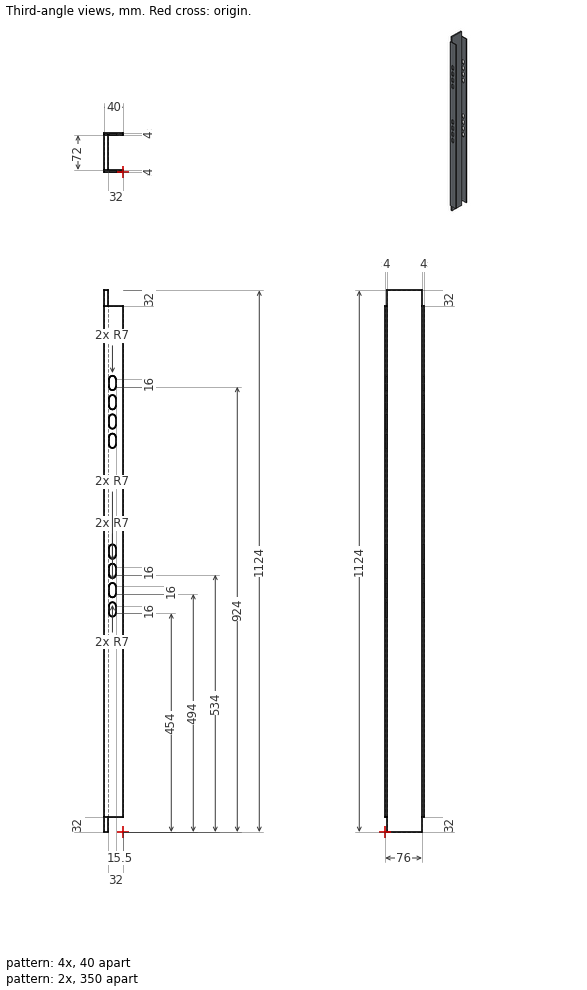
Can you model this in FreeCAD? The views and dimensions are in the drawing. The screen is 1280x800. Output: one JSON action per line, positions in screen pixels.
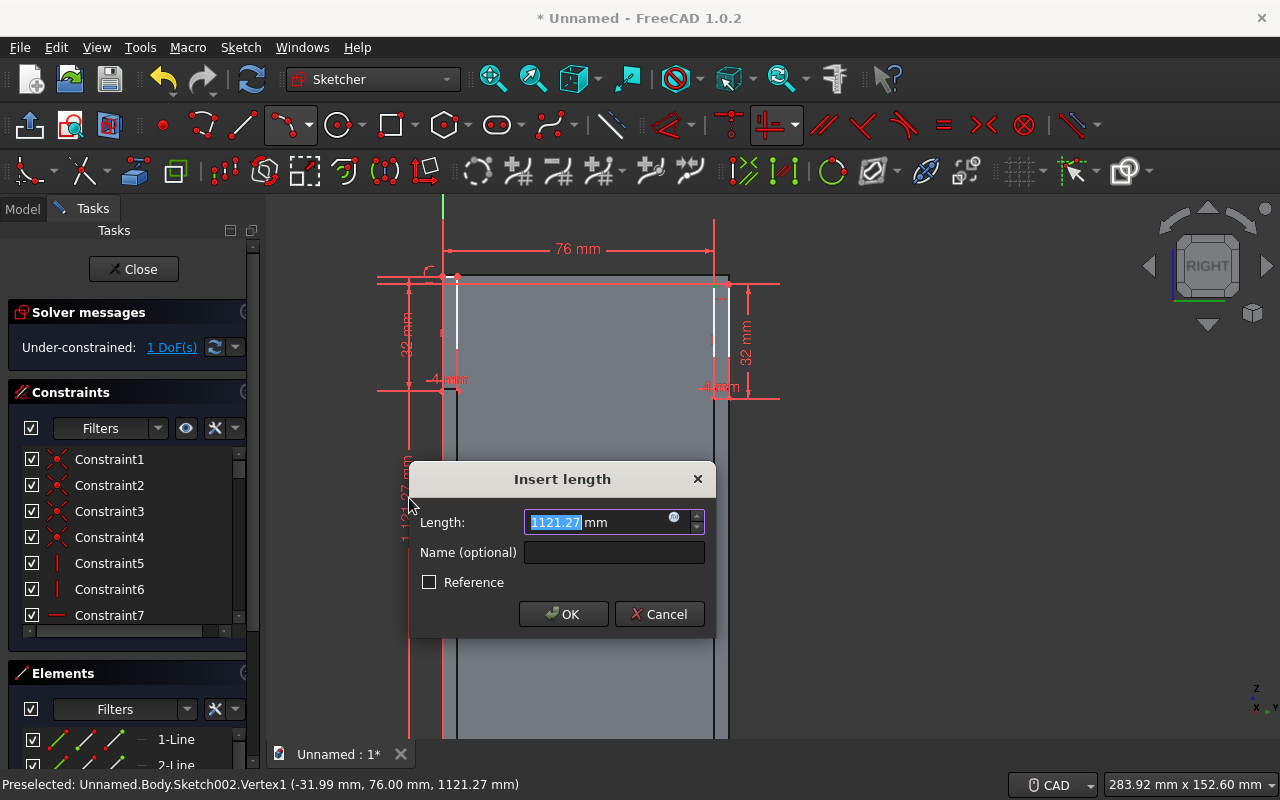
{"action": "type", "text": "1124"}
{"action": "key", "text": "Return"}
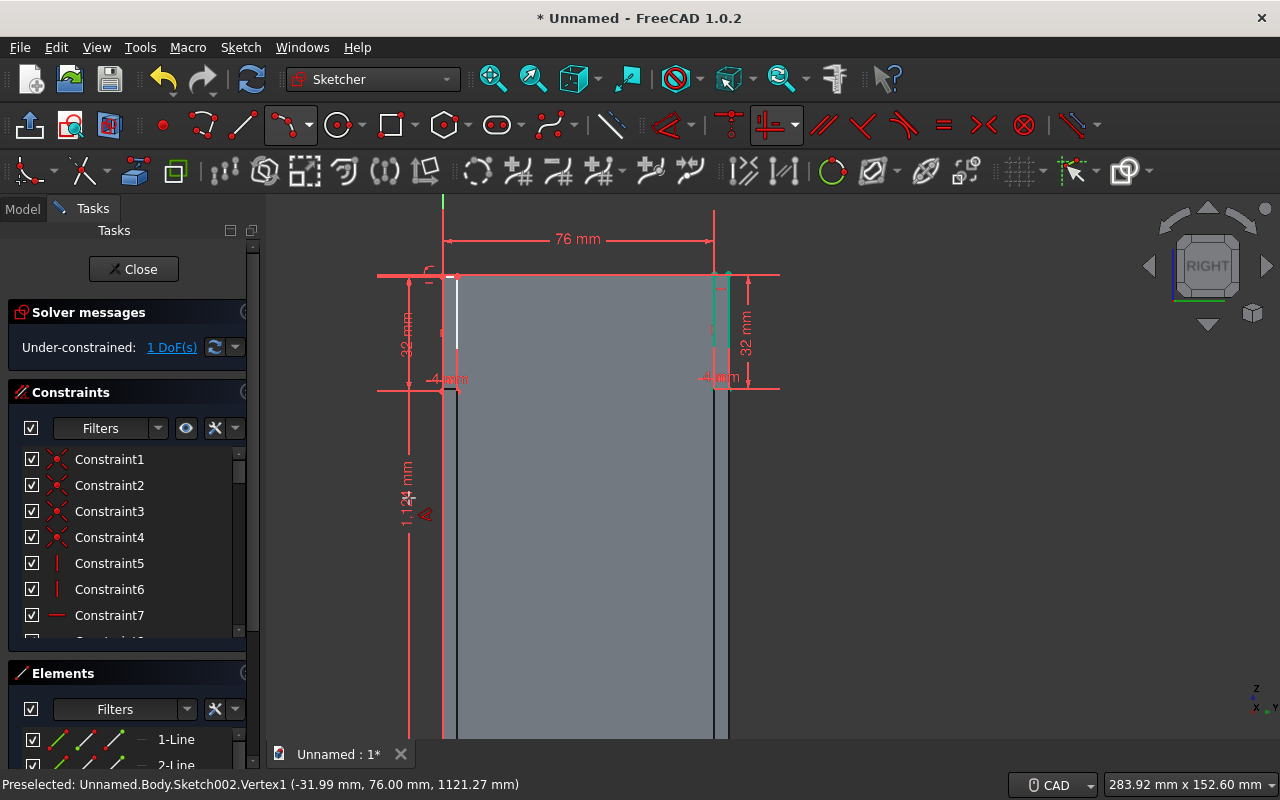
{"action": "left_click", "coordinate": [443, 277]}
{"action": "left_click", "coordinate": [409, 594]}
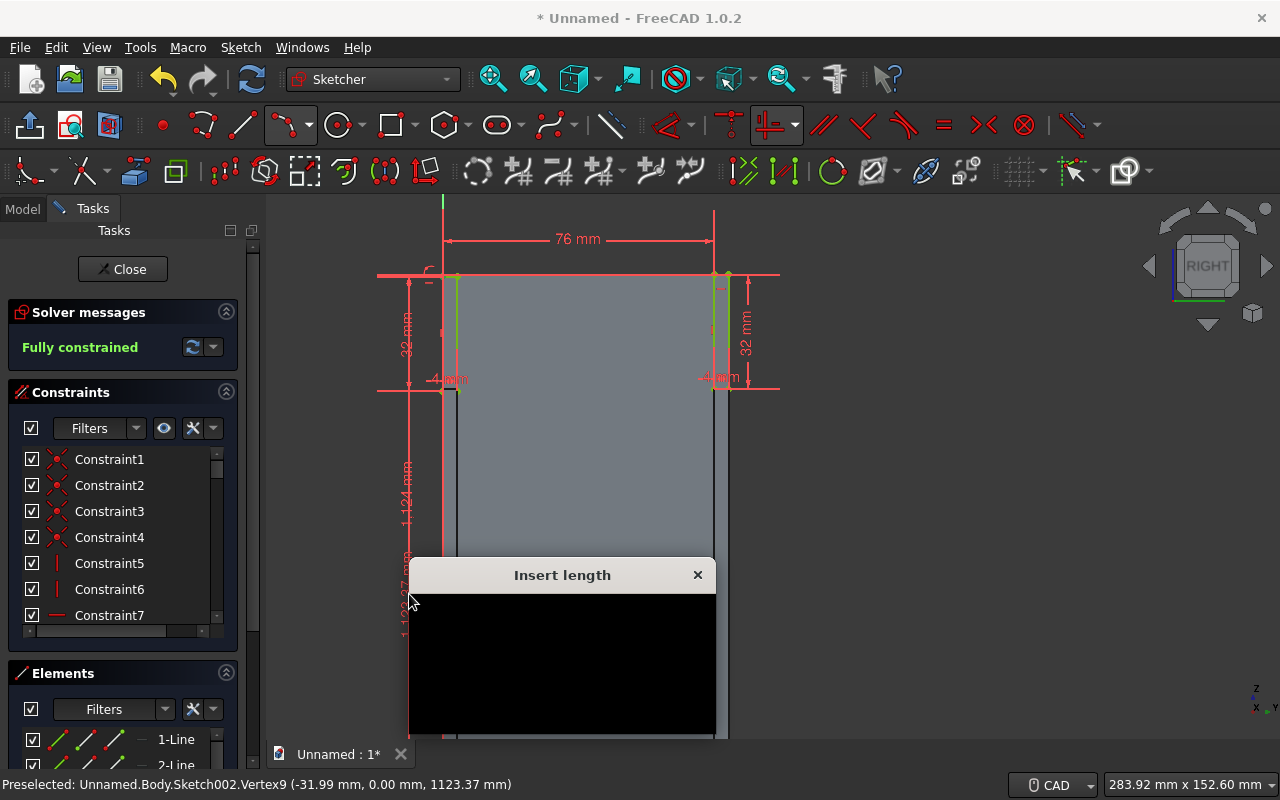
{"action": "type", "text": "1124"}
{"action": "key", "text": "Return"}
{"action": "key", "text": "Escape"}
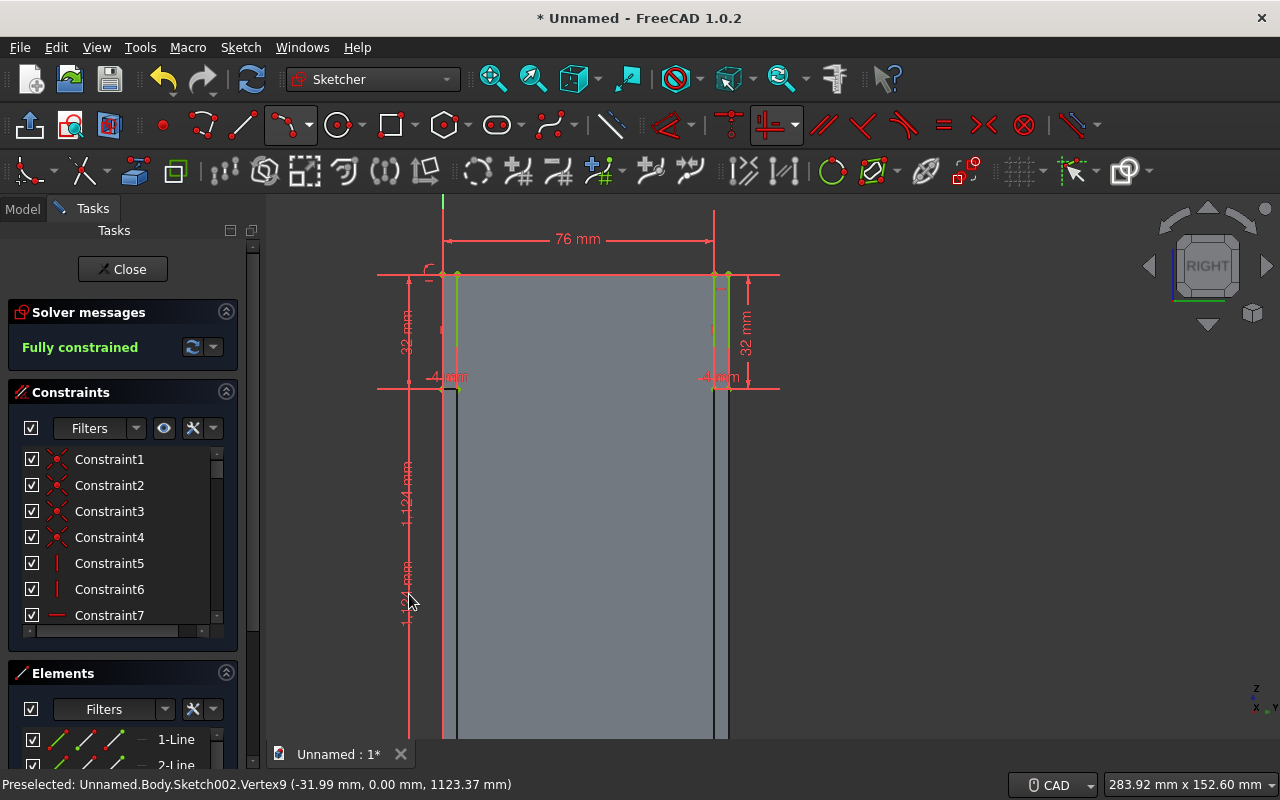
{"action": "left_click", "coordinate": [123, 269]}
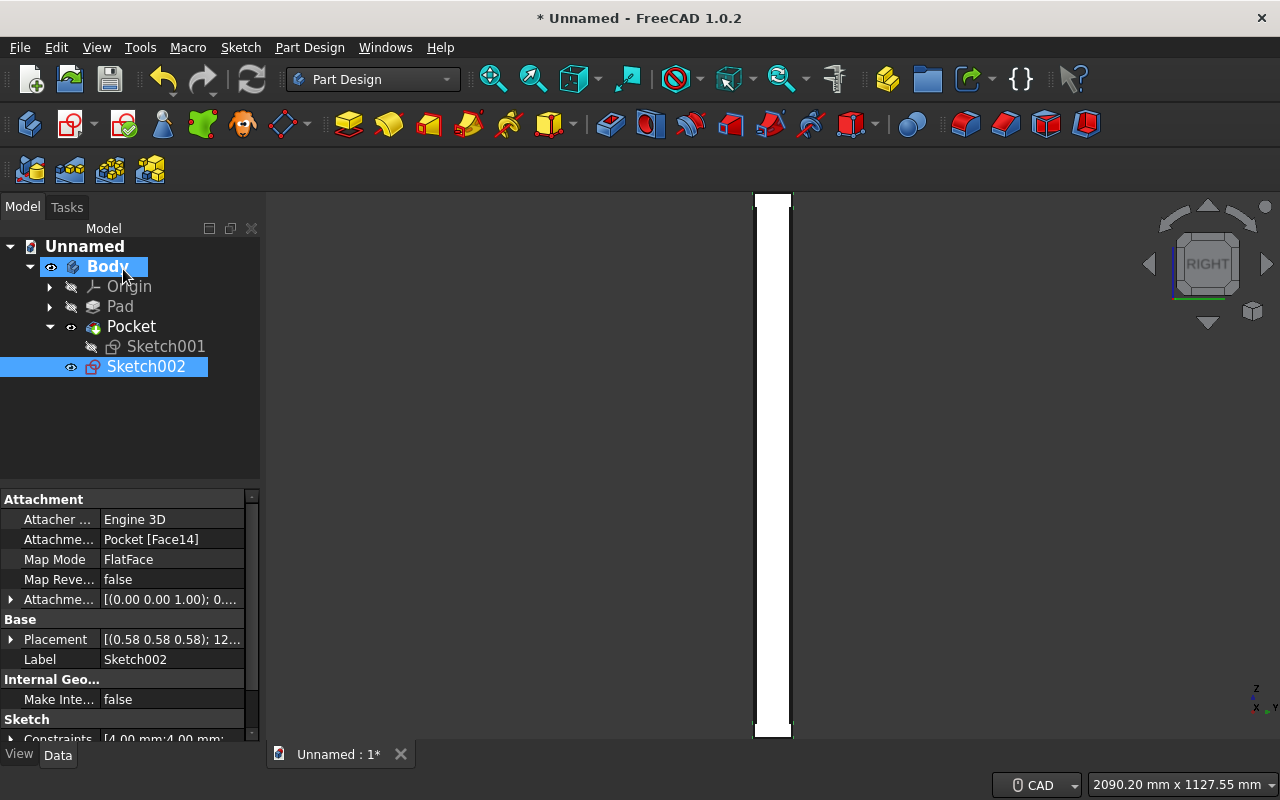
{"action": "left_click", "coordinate": [612, 124]}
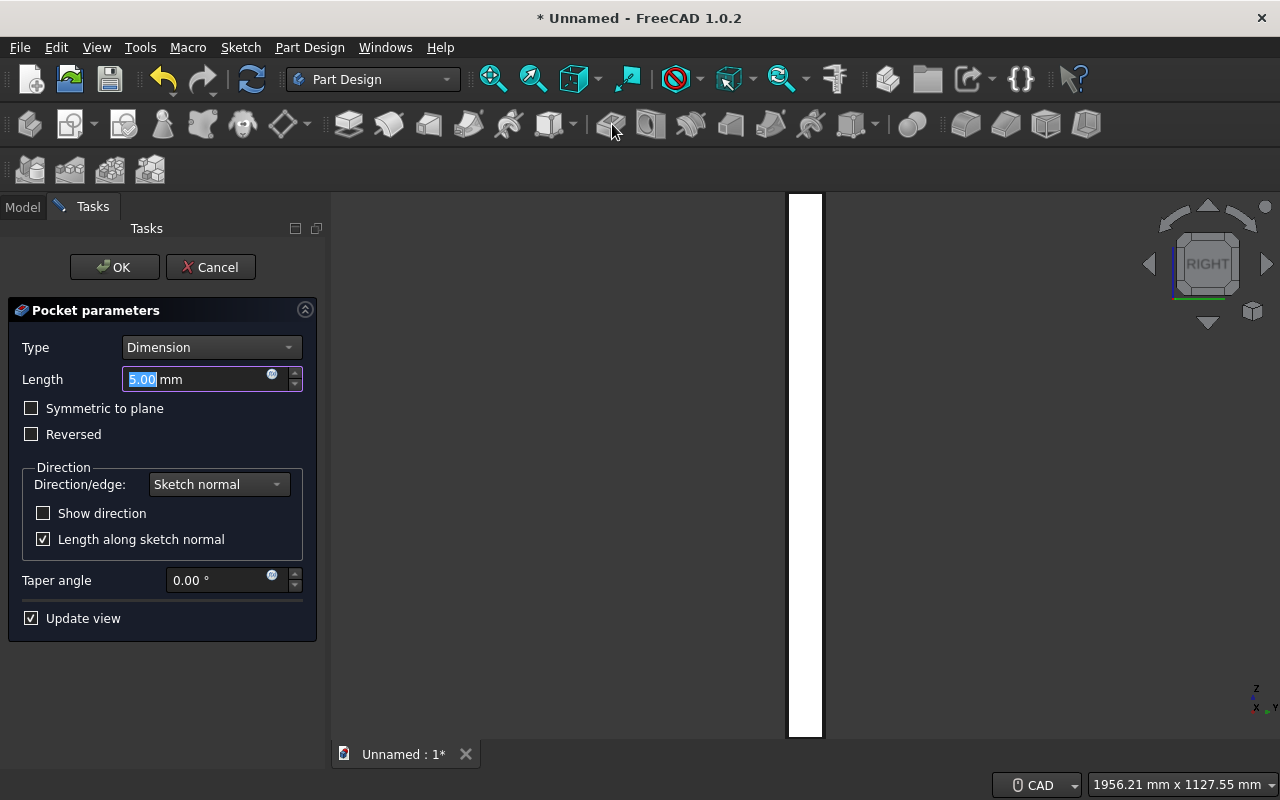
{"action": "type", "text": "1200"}
{"action": "key", "text": "Tab"}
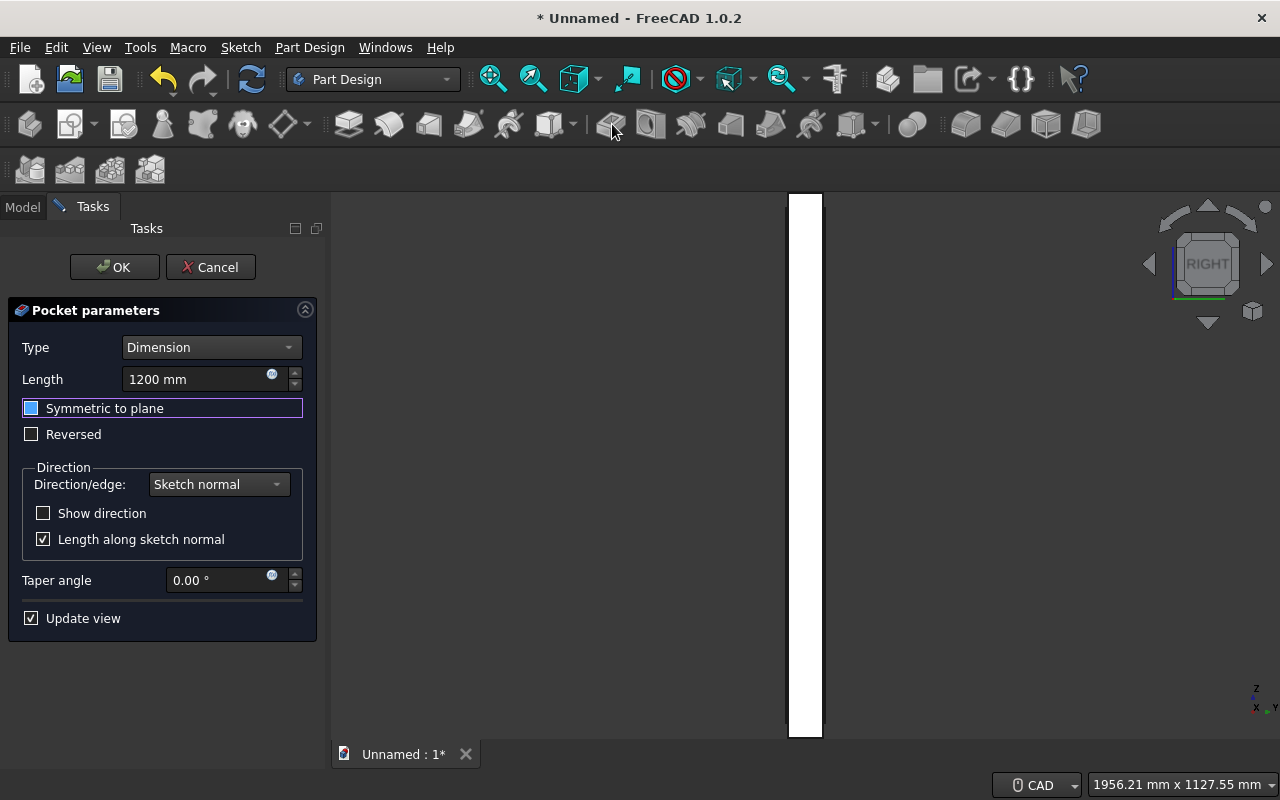
{"action": "left_click", "coordinate": [115, 267]}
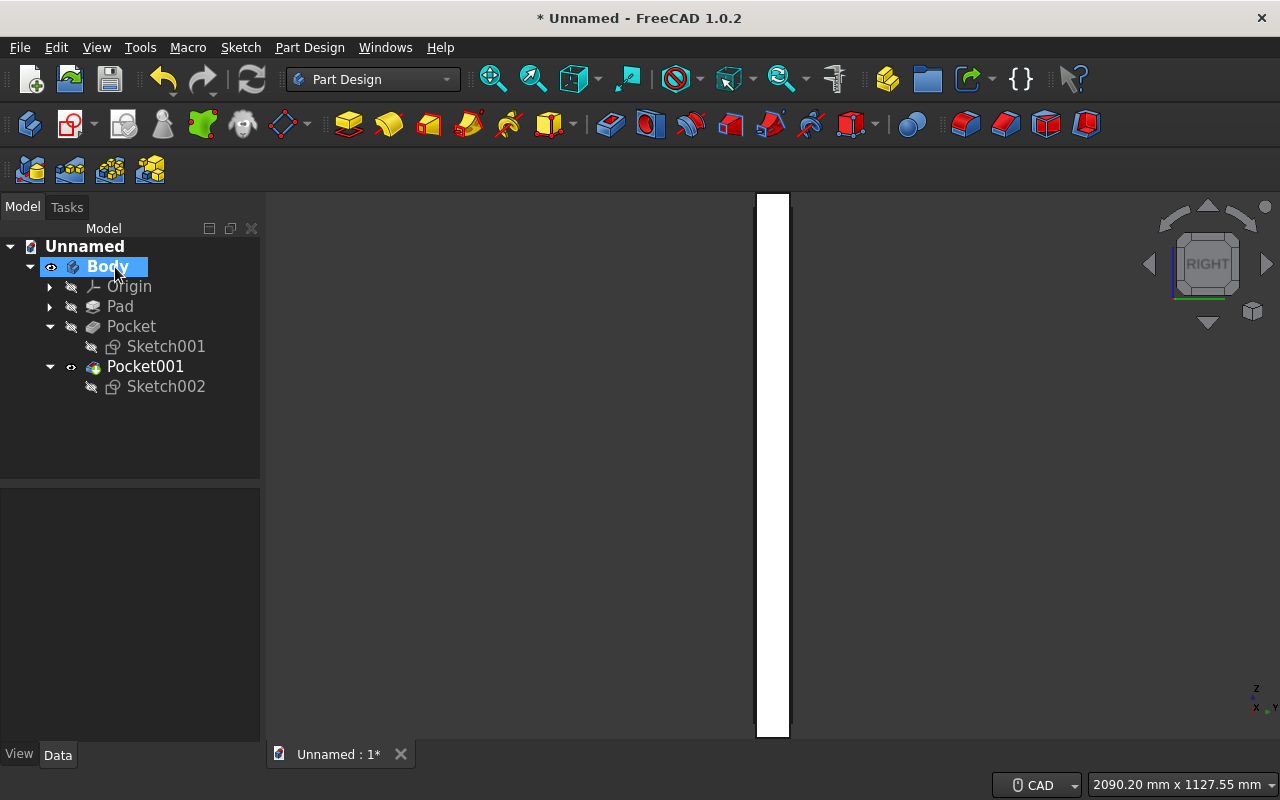
{"action": "key", "text": "4"}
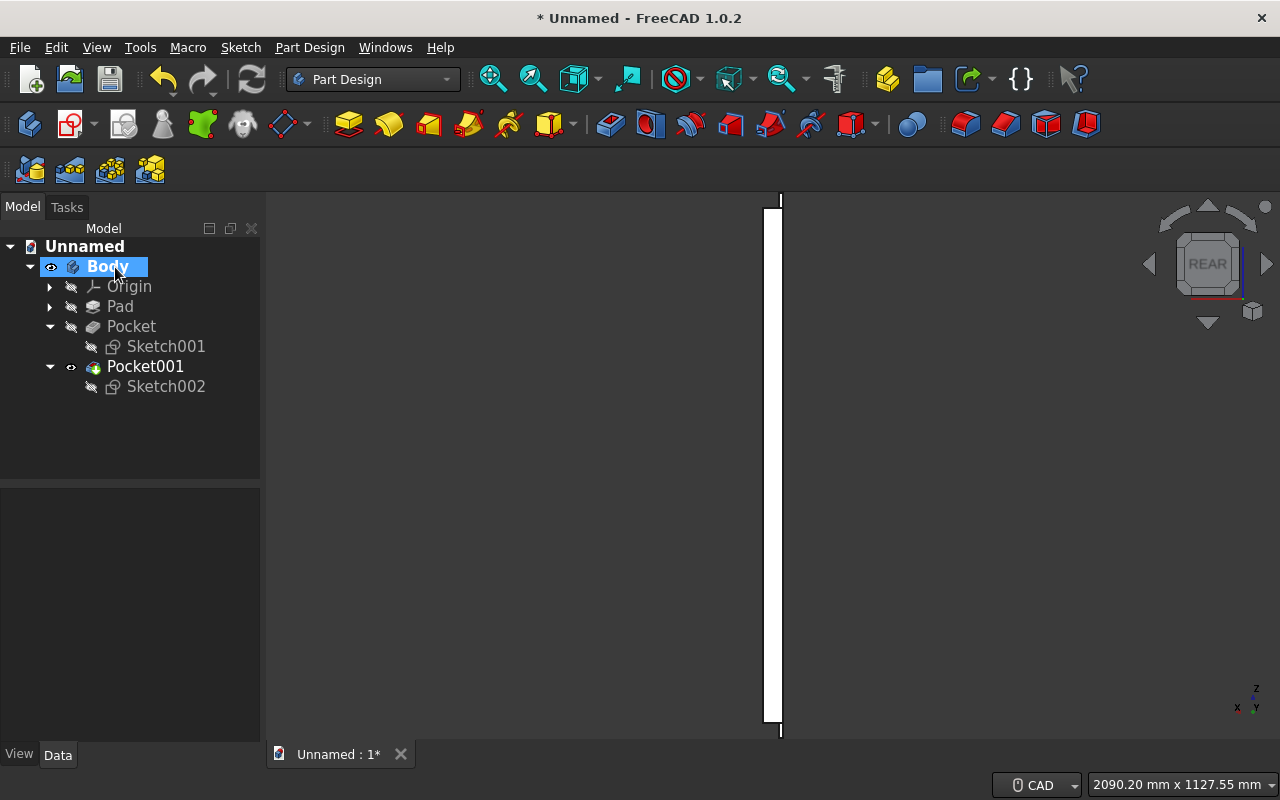
{"action": "left_click", "coordinate": [773, 244]}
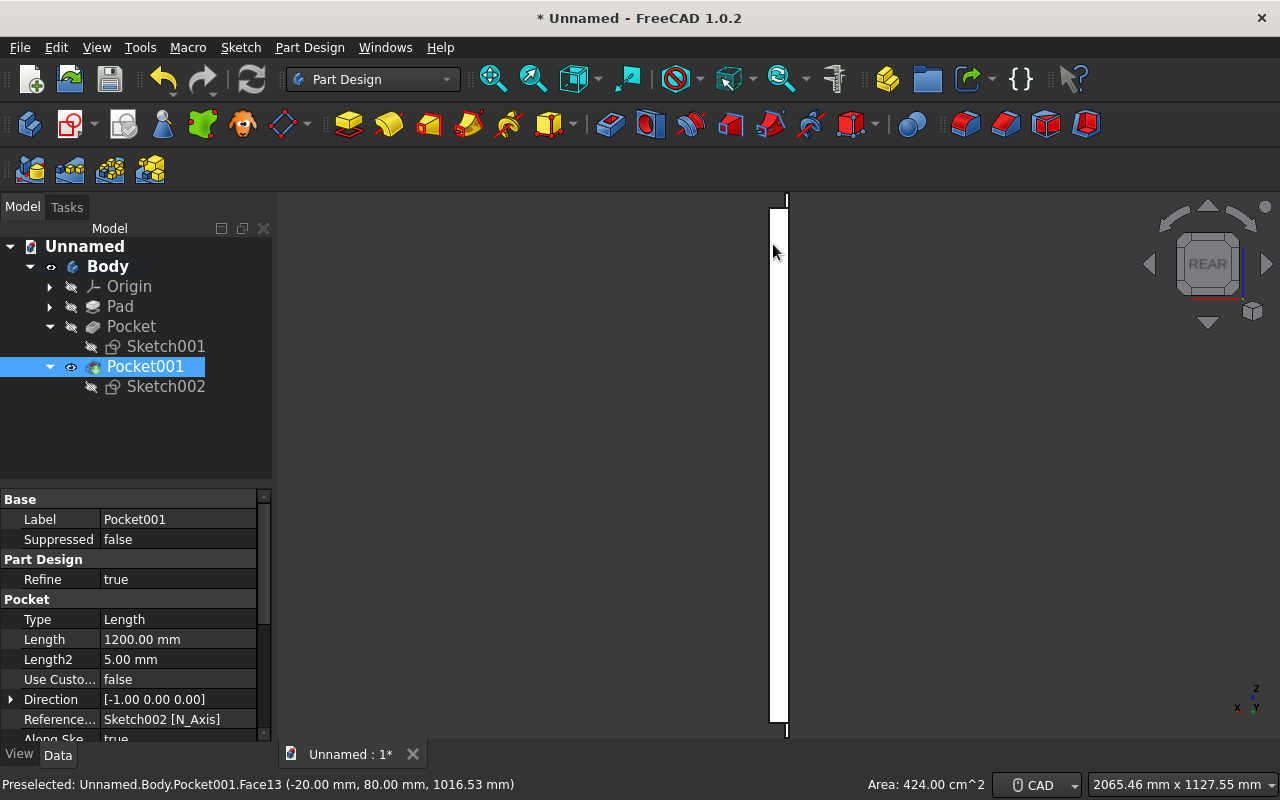
{"action": "left_click", "coordinate": [70, 124]}